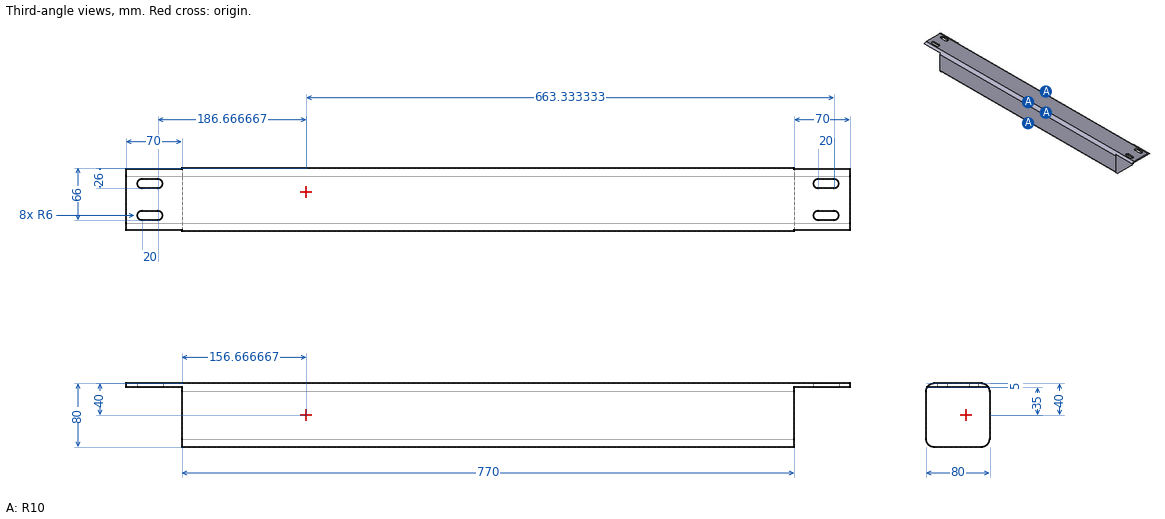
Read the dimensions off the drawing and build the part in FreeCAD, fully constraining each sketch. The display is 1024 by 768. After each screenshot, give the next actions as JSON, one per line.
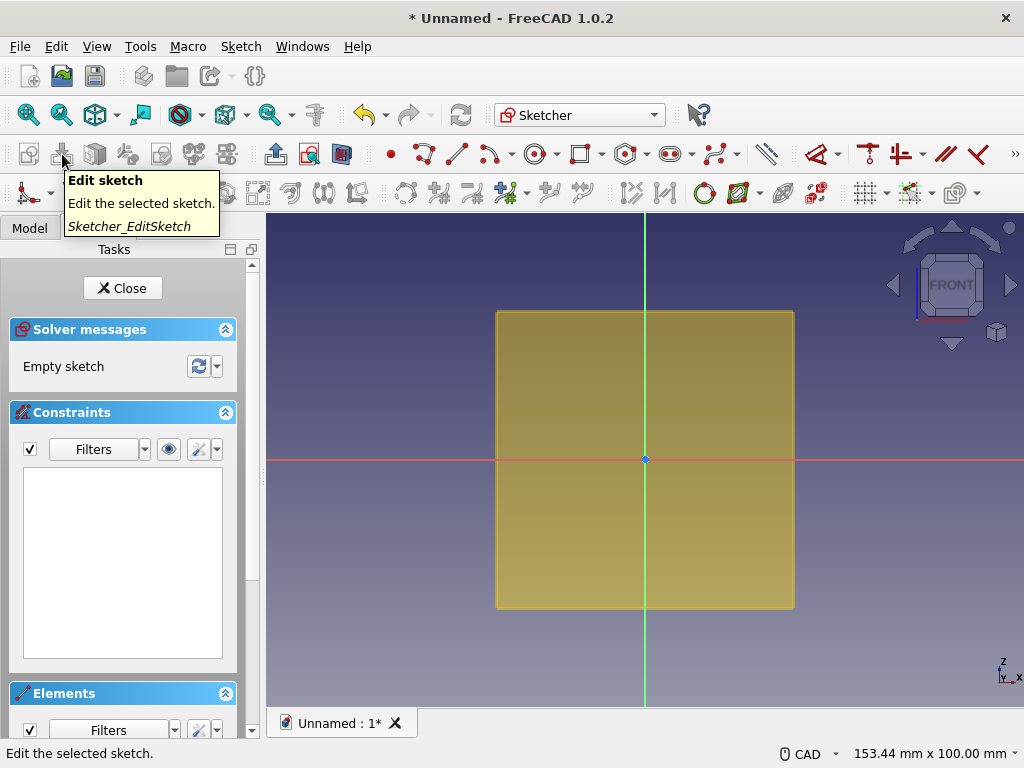
{"action": "scroll", "coordinate": [427, 460], "scroll_direction": "down", "scroll_amount": 11}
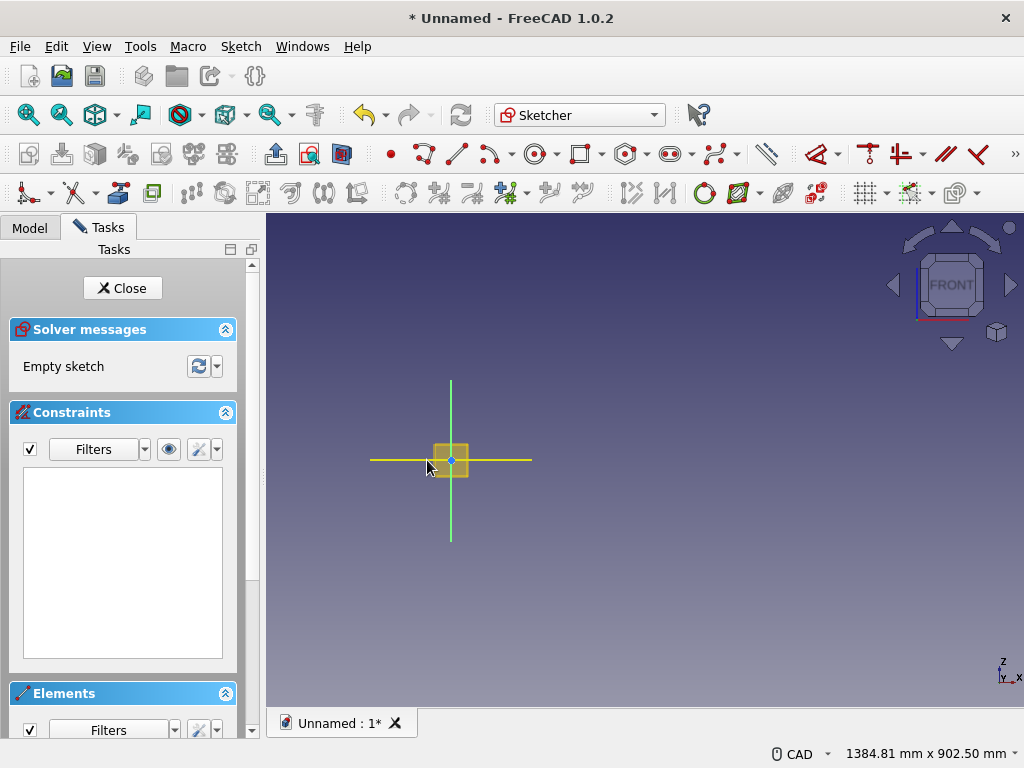
{"action": "left_click", "coordinate": [580, 154]}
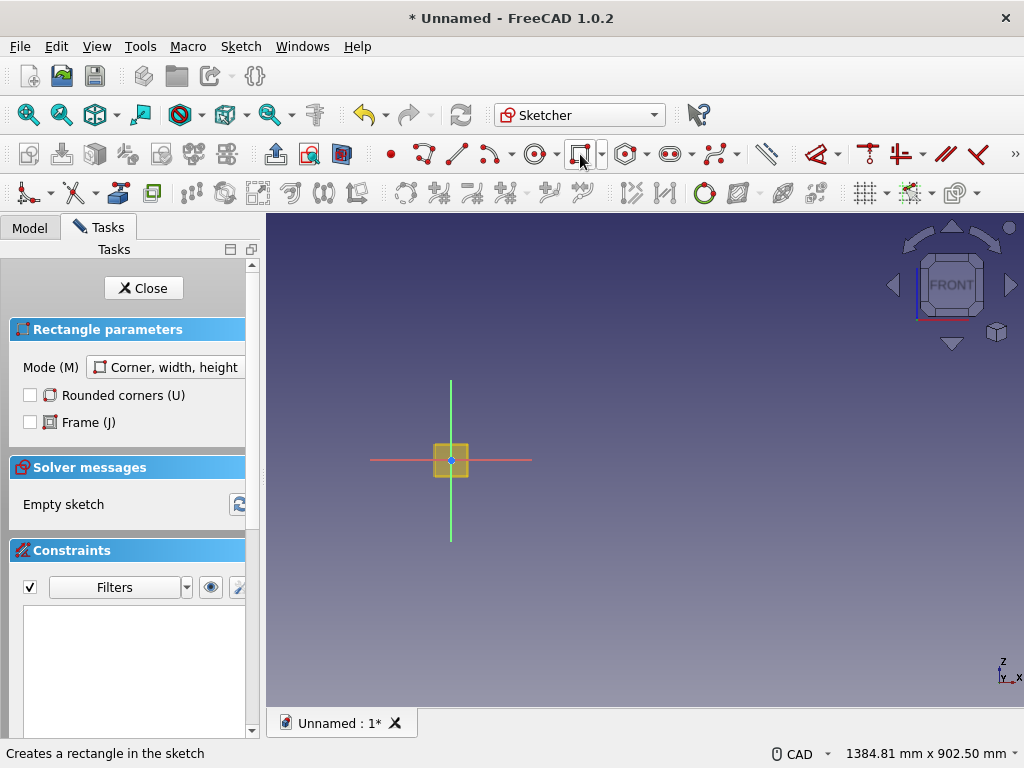
{"action": "left_click", "coordinate": [366, 439]}
{"action": "left_click", "coordinate": [787, 482]}
{"action": "key", "text": "Escape"}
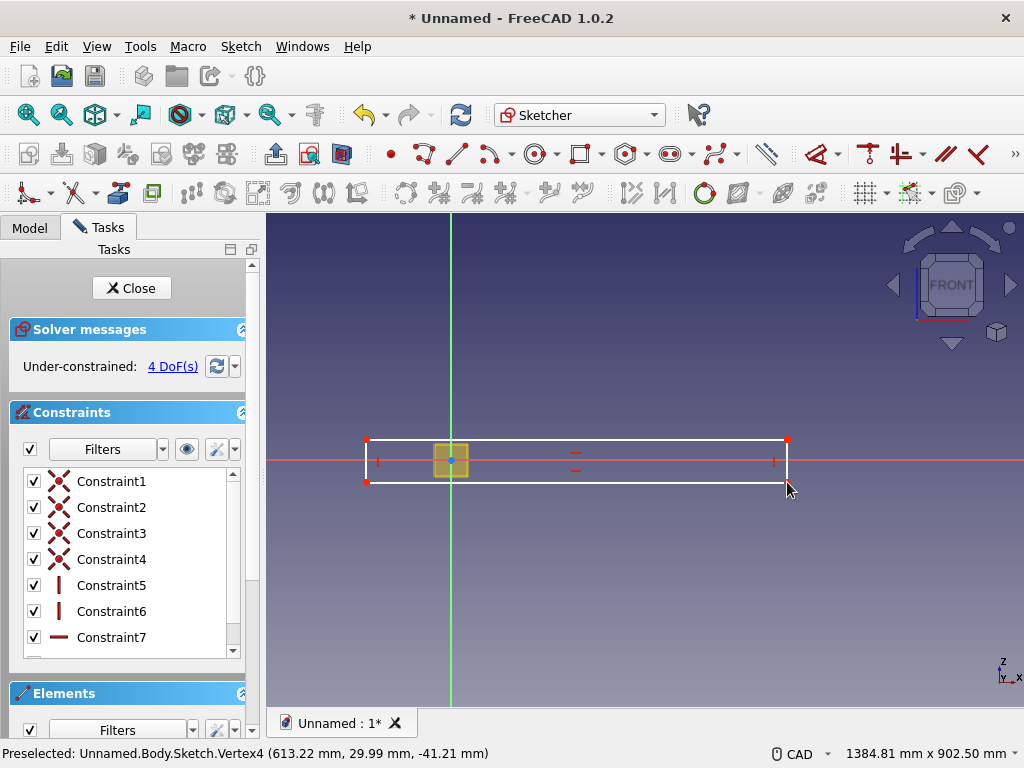
{"action": "scroll", "coordinate": [366, 470], "scroll_direction": "up", "scroll_amount": 2}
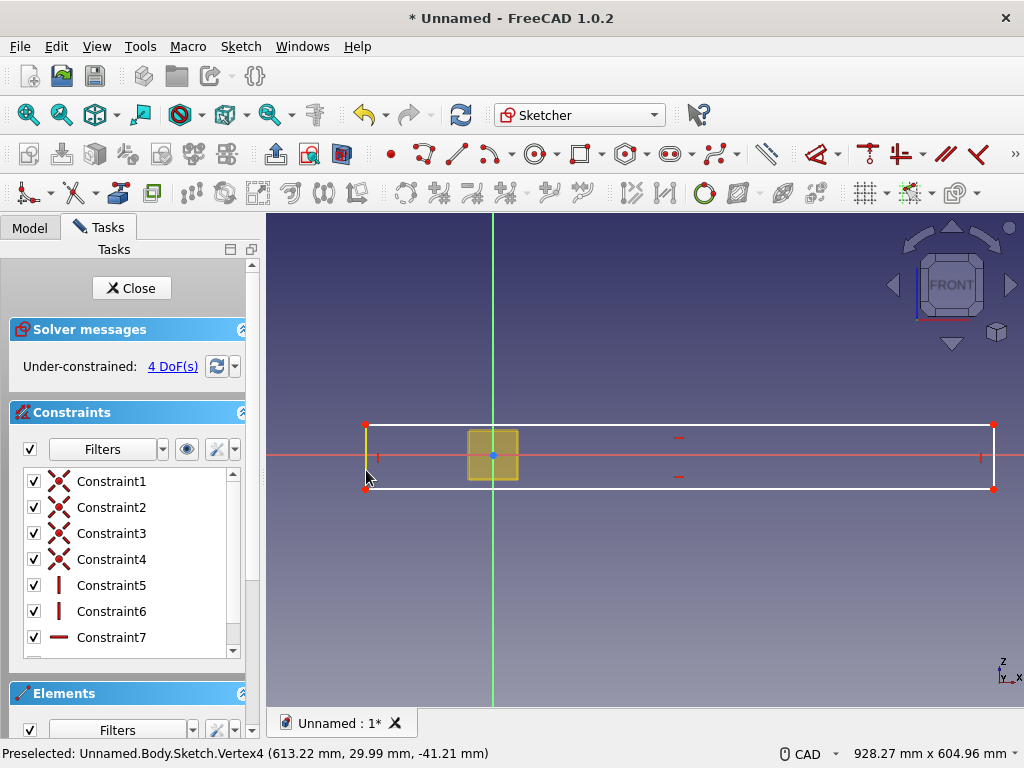
{"action": "left_click", "coordinate": [366, 470]}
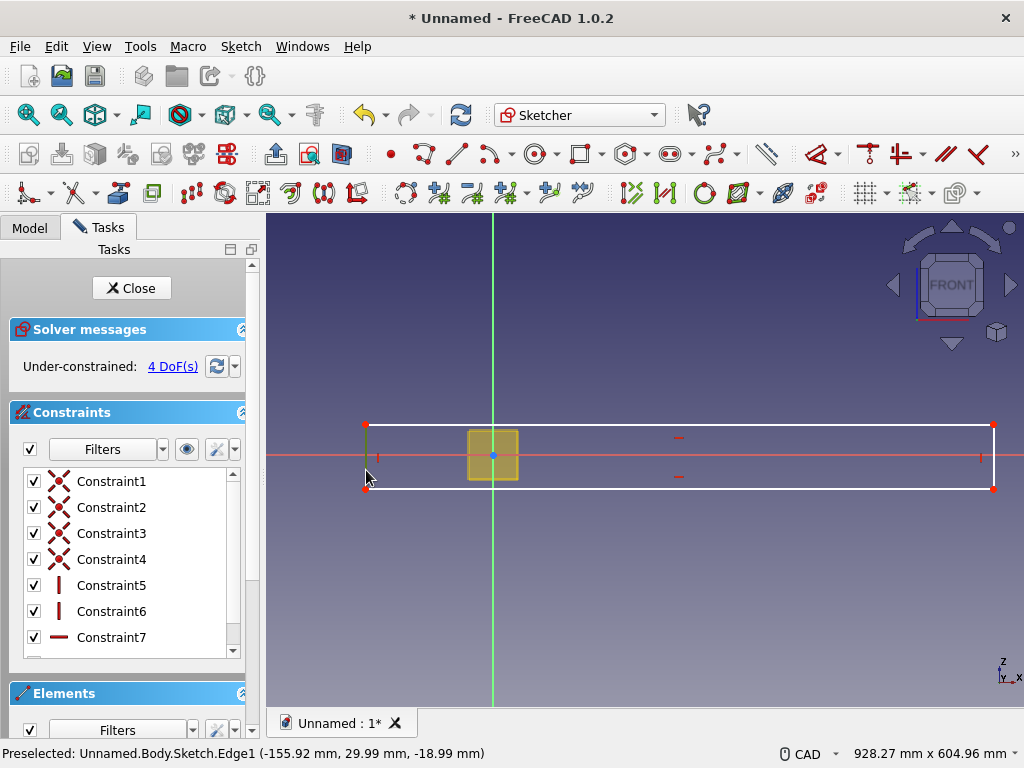
{"action": "left_click", "coordinate": [838, 154]}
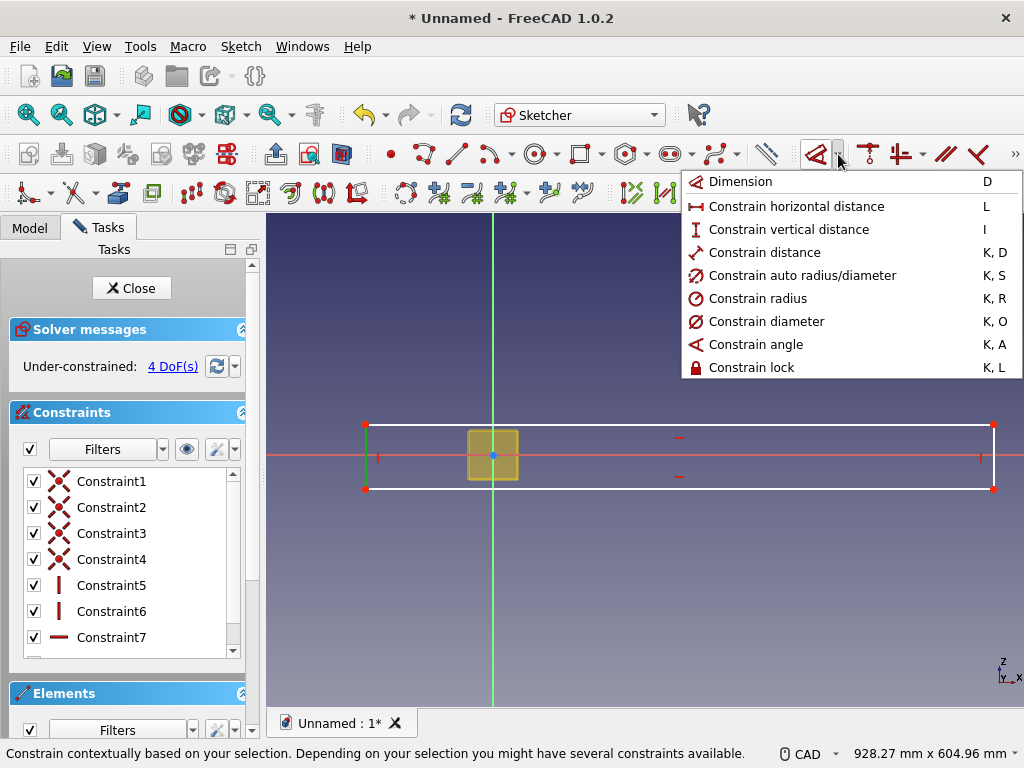
{"action": "left_click", "coordinate": [852, 230]}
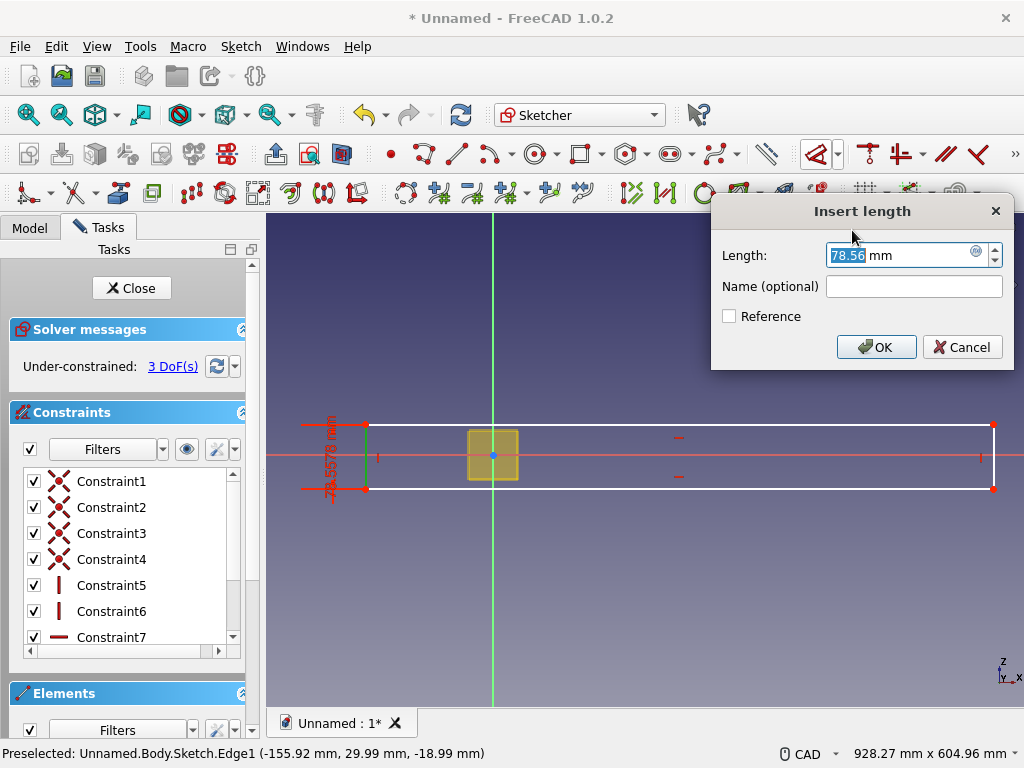
{"action": "type", "text": "80"}
{"action": "key", "text": "Return"}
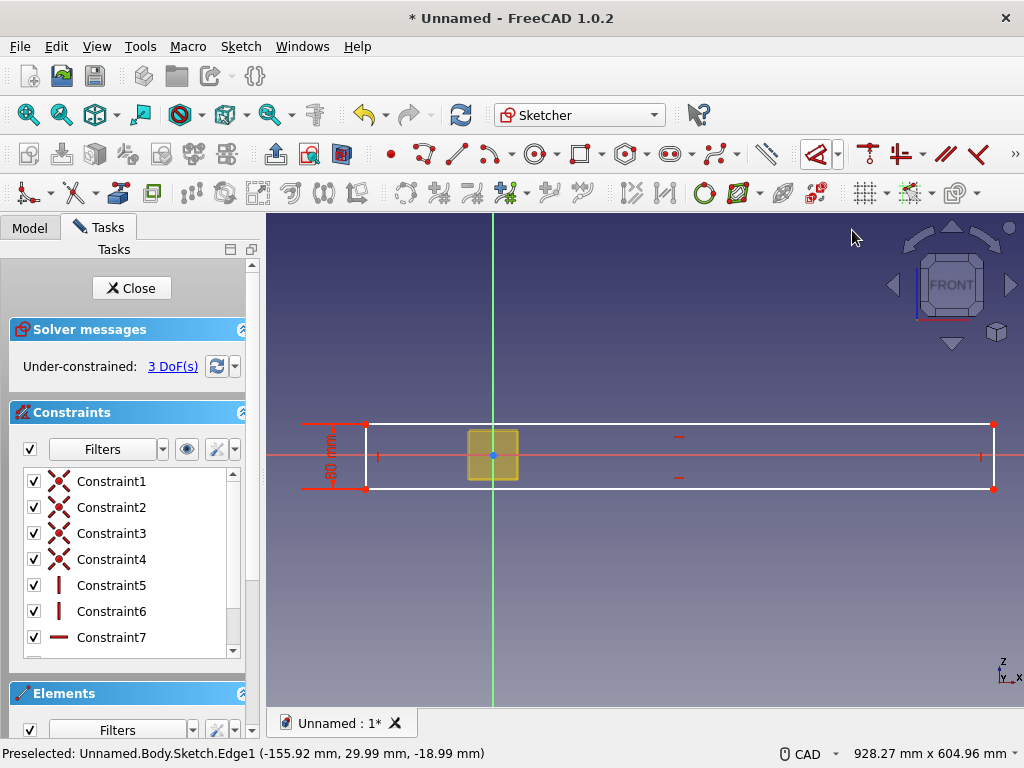
{"action": "left_click", "coordinate": [554, 489]}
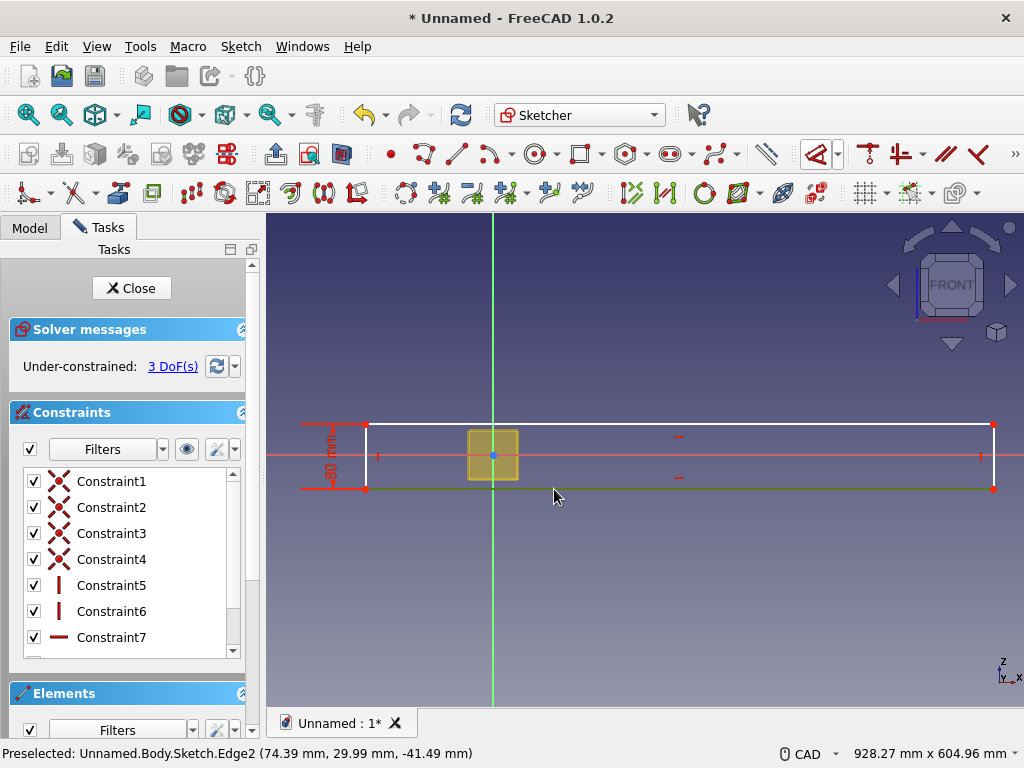
{"action": "key", "text": "l"}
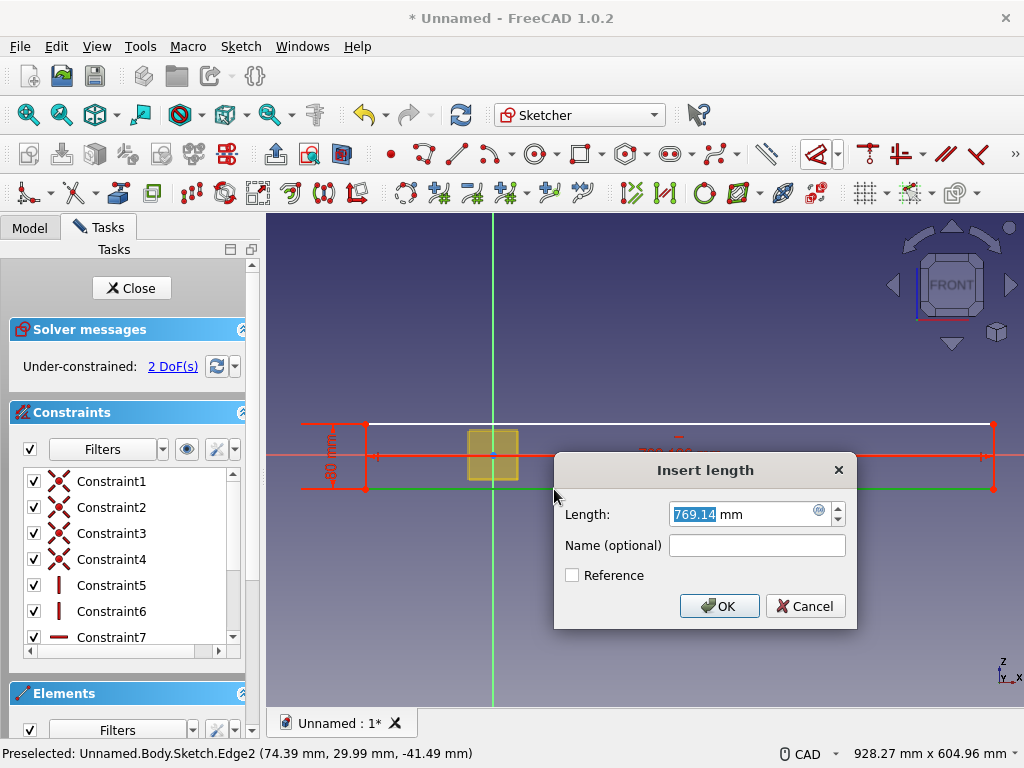
{"action": "type", "text": "770"}
{"action": "key", "text": "Return"}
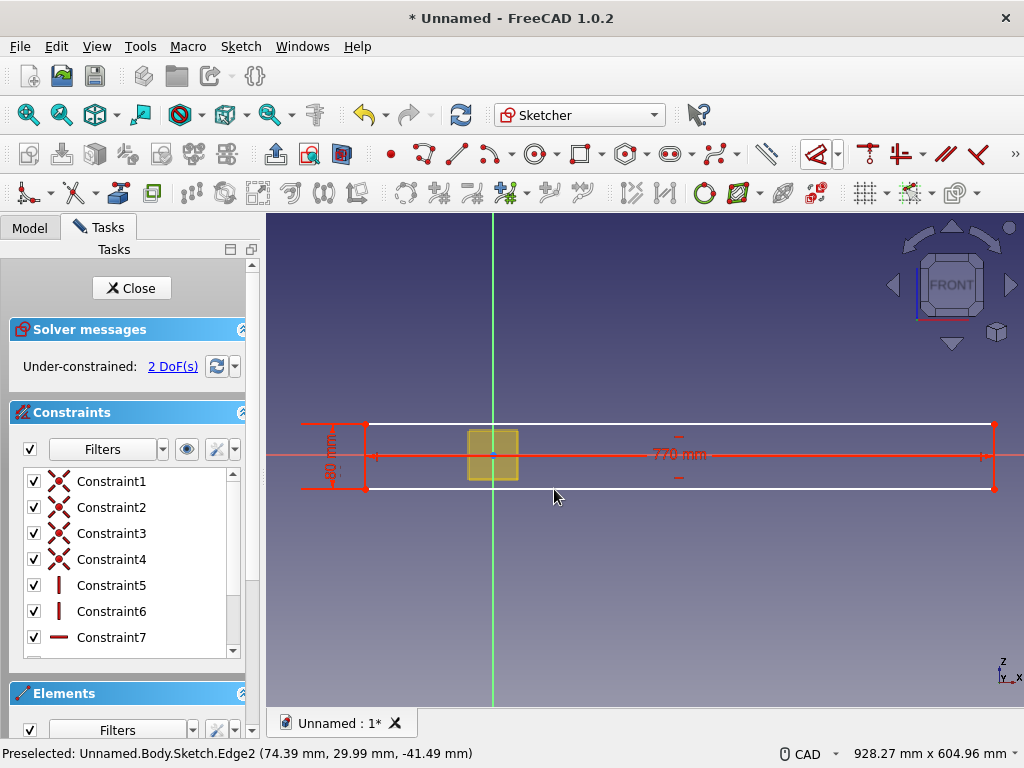
{"action": "left_click", "coordinate": [365, 424]}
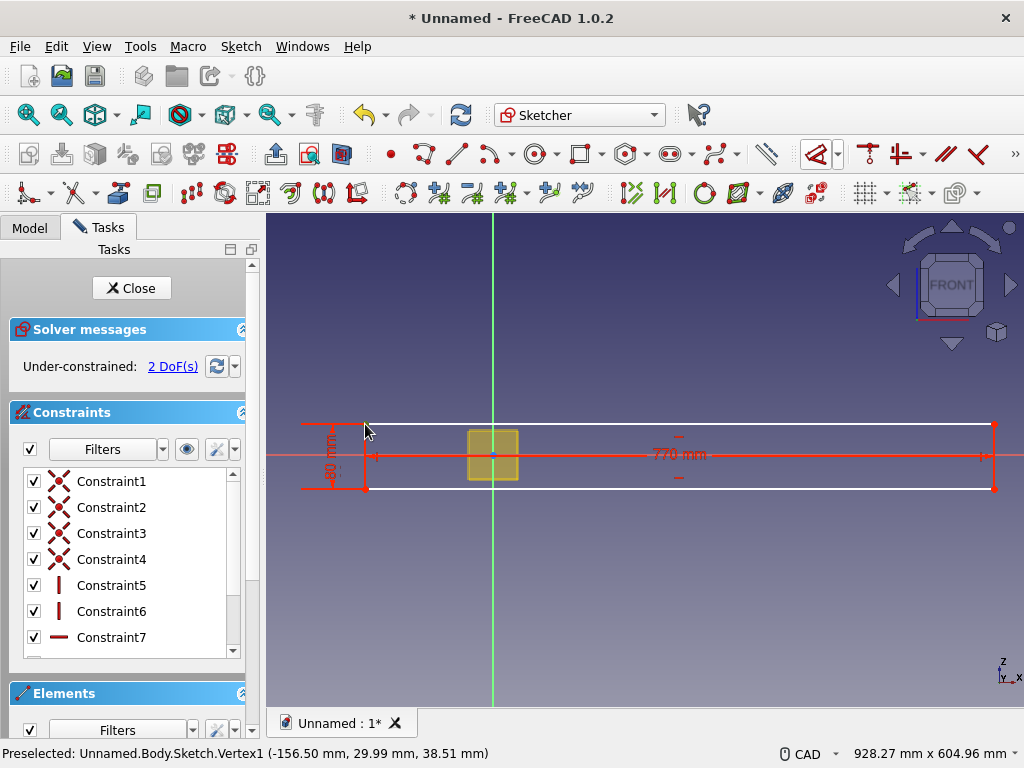
{"action": "key", "text": "i"}